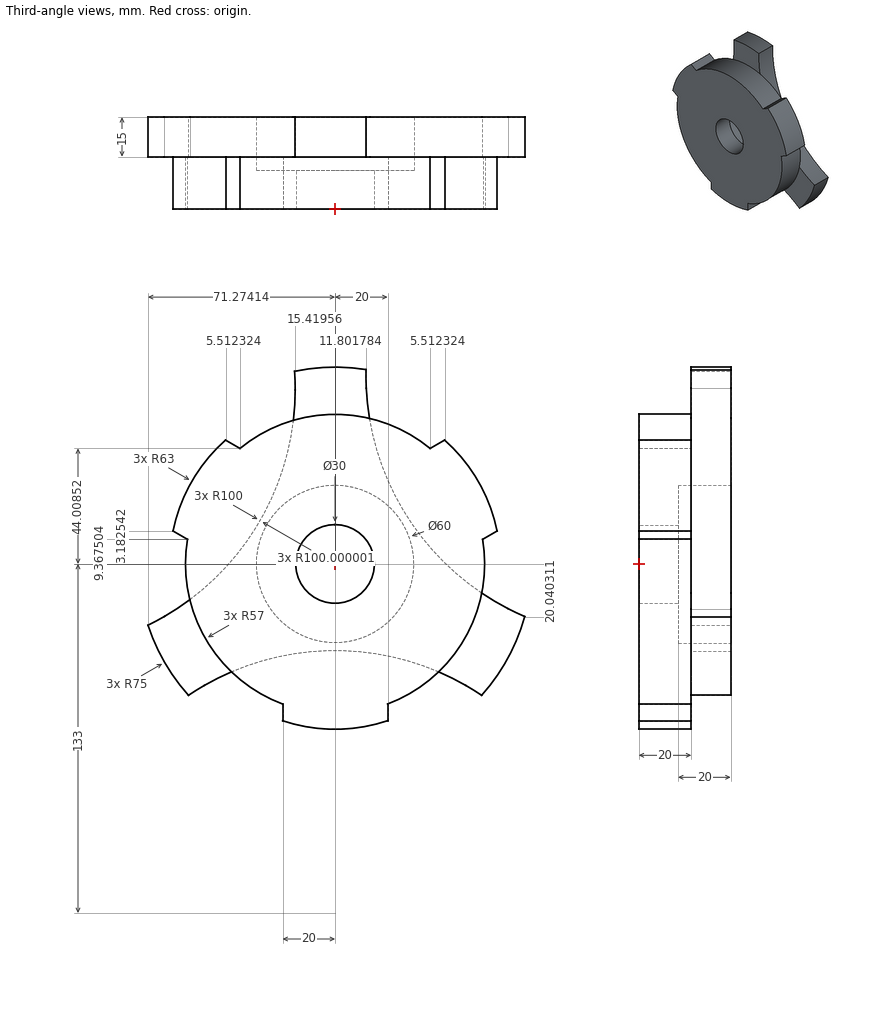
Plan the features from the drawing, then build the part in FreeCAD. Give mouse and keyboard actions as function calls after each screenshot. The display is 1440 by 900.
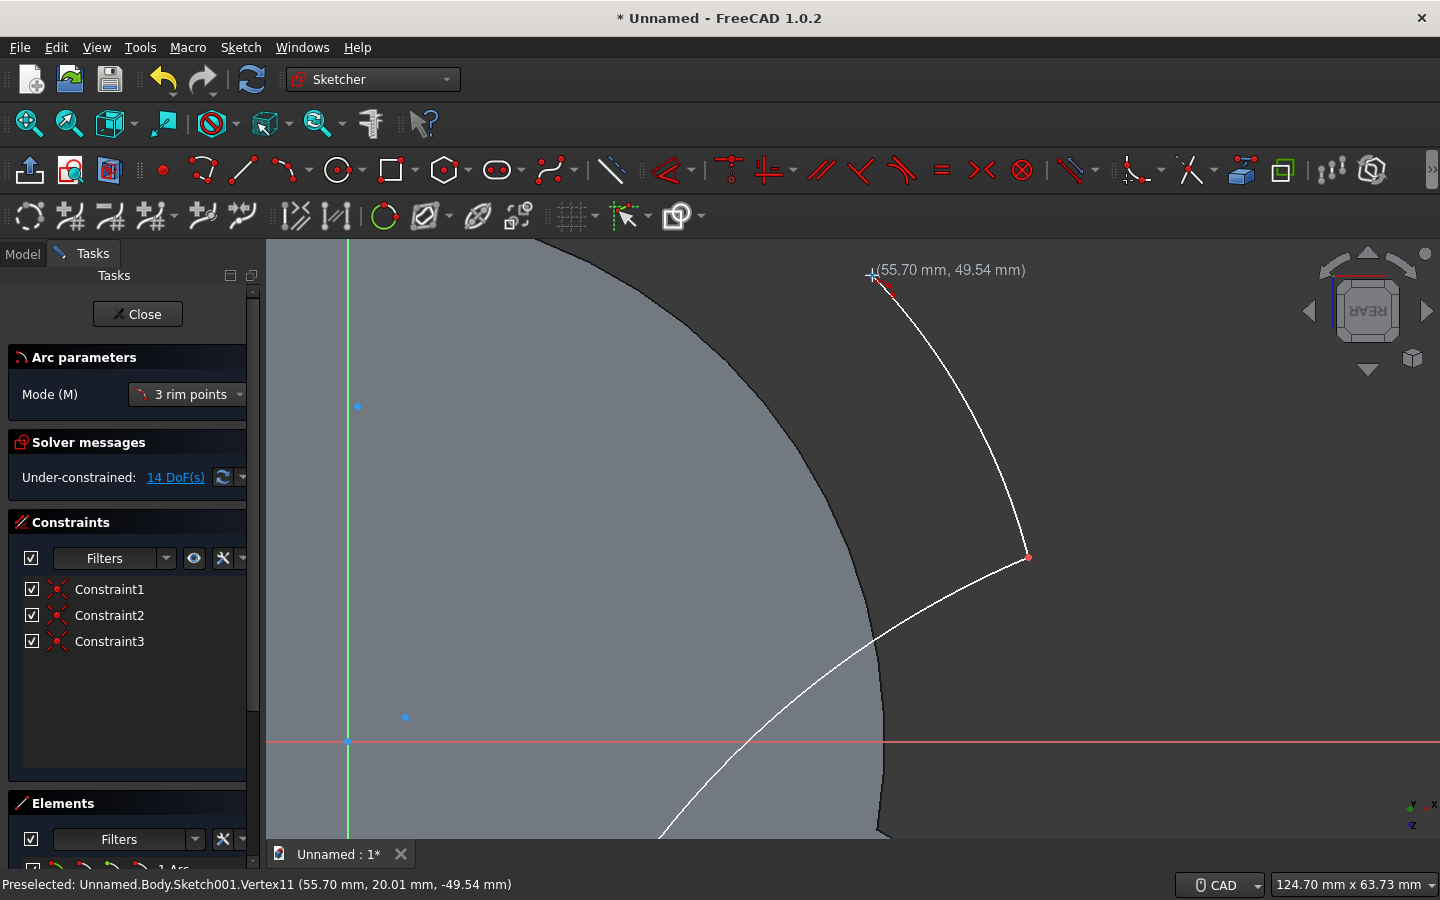
scroll(971, 401, down, 6)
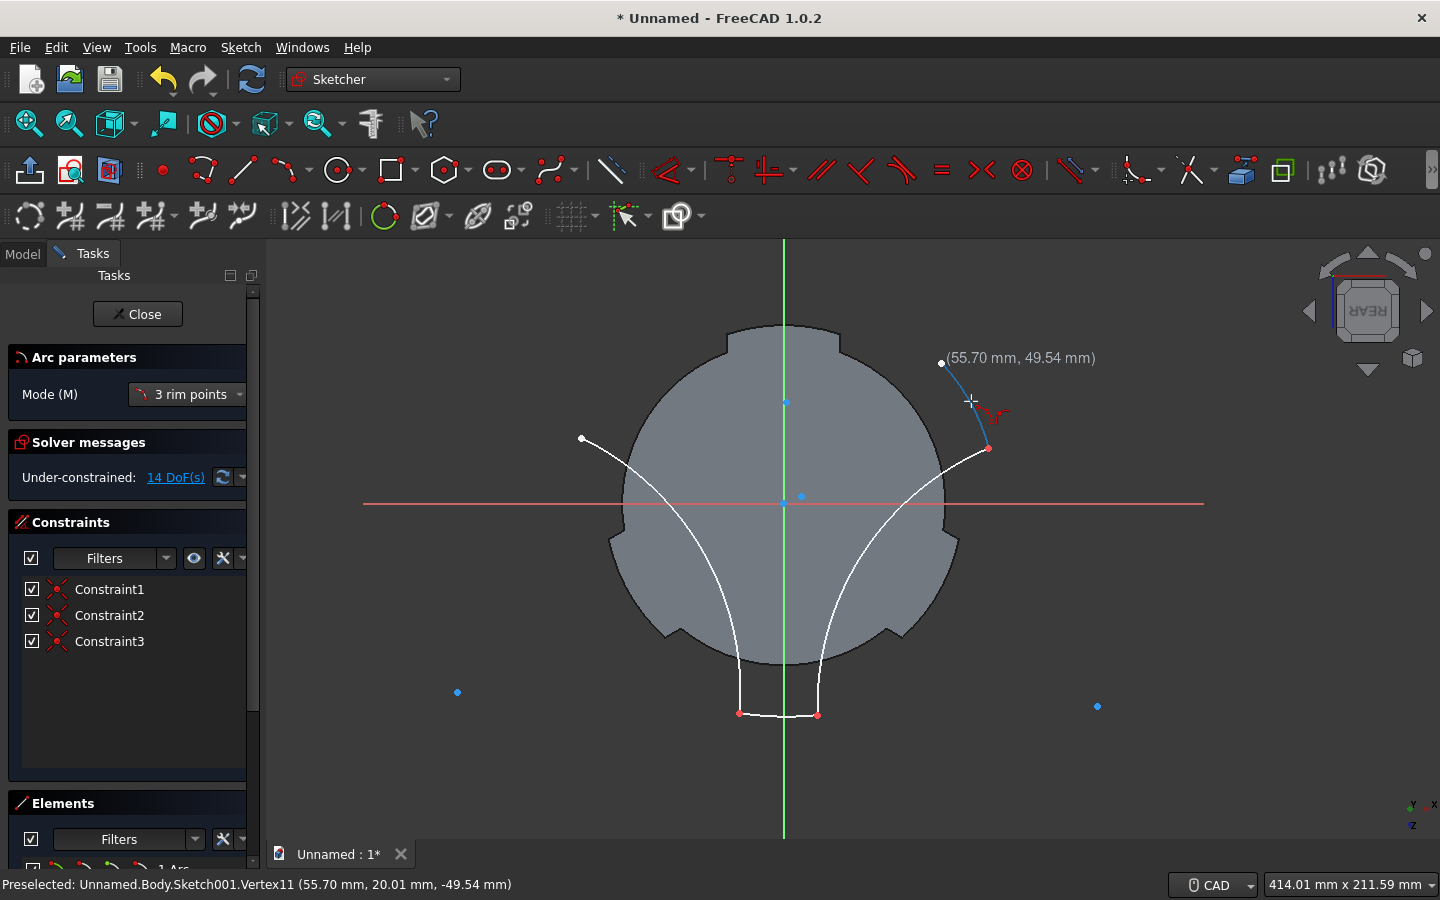
click(625, 362)
click(750, 408)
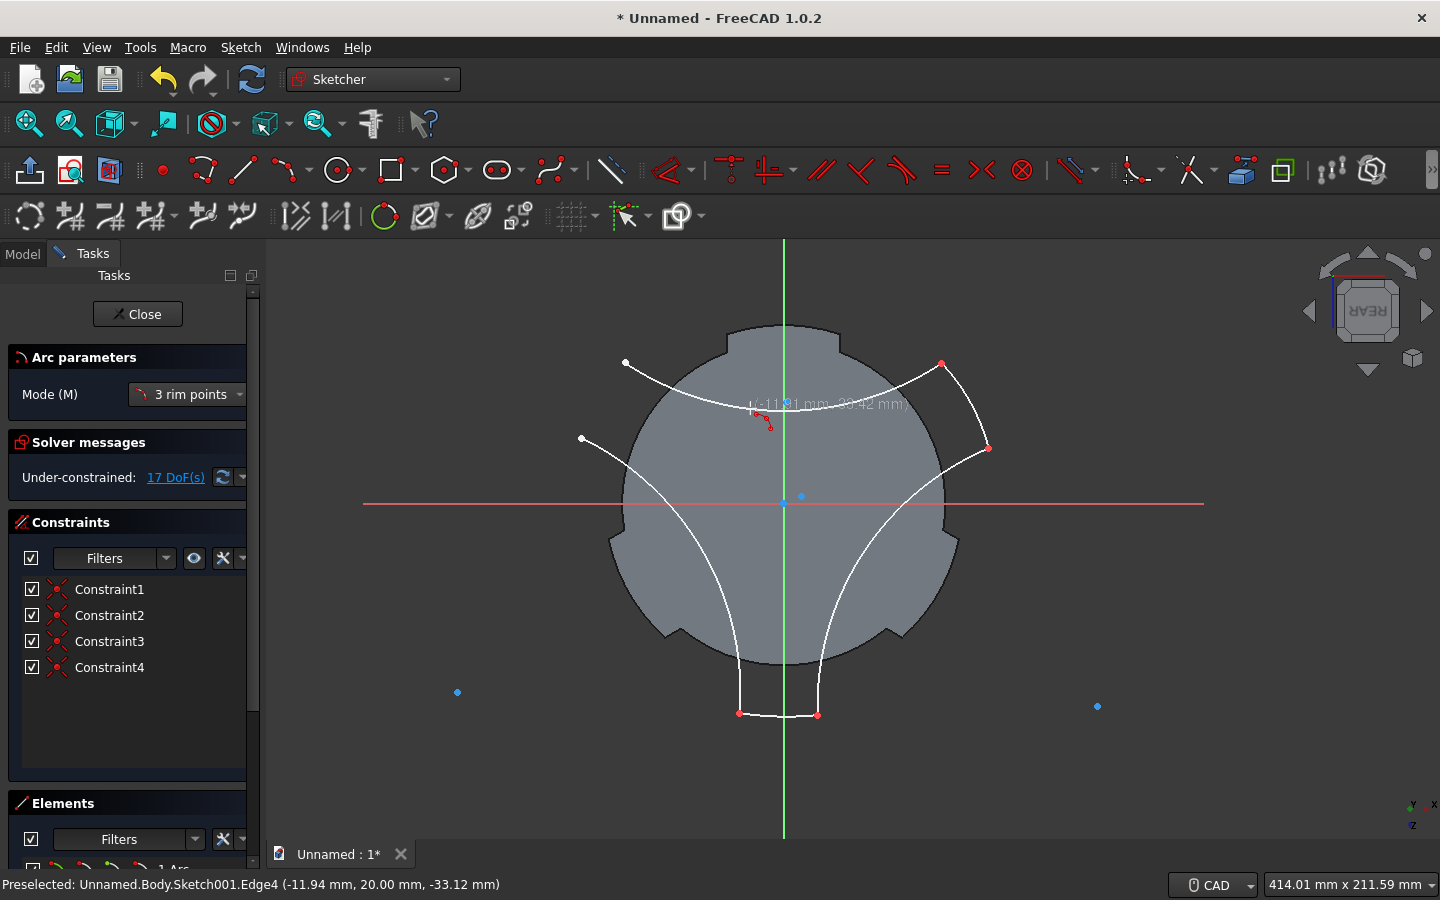
click(625, 363)
click(582, 438)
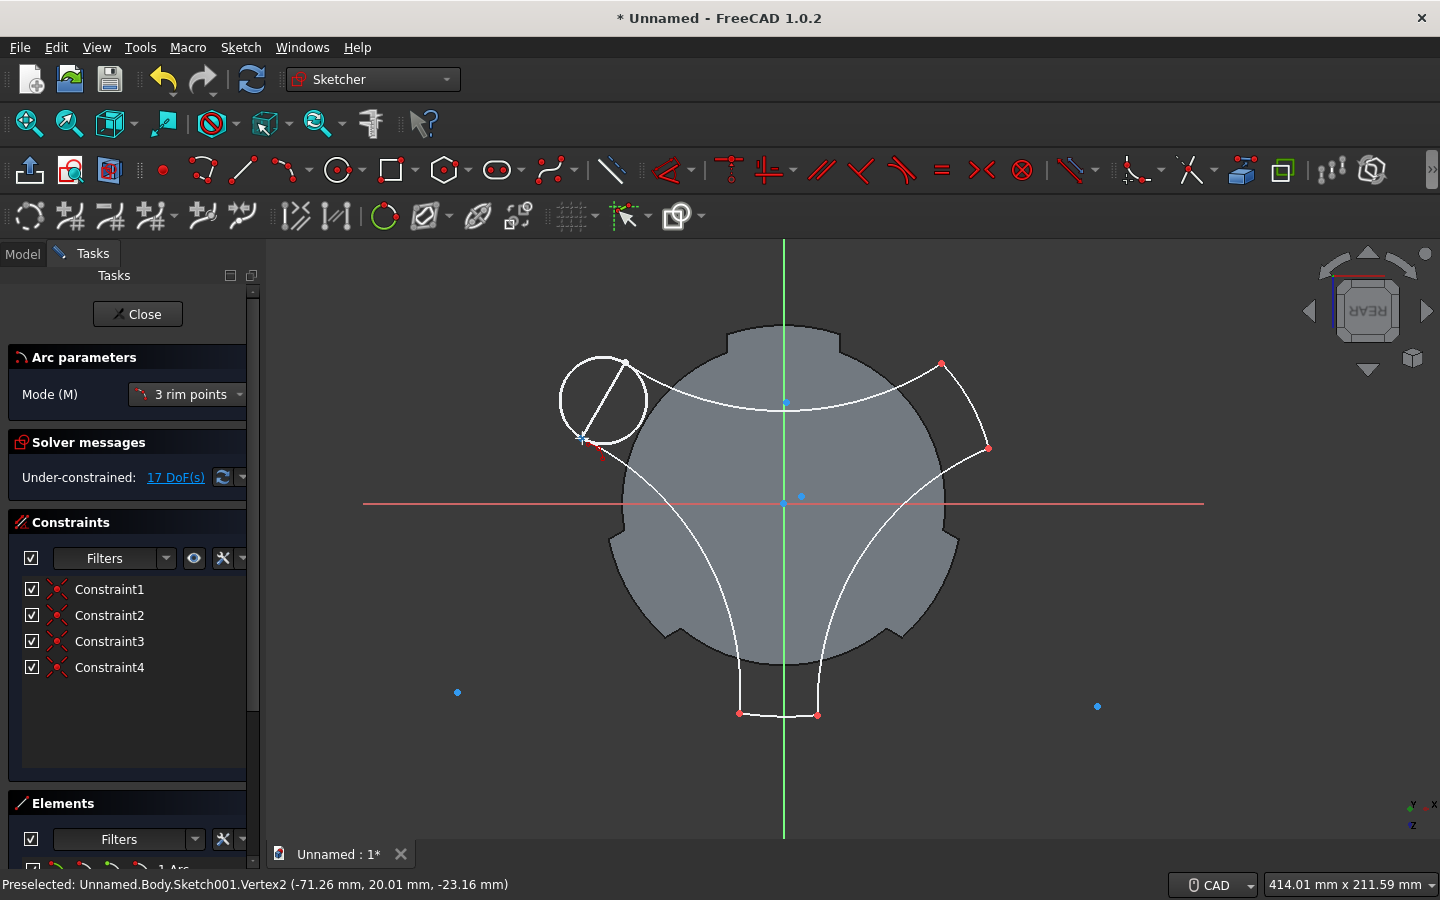
scroll(600, 397, up, 7)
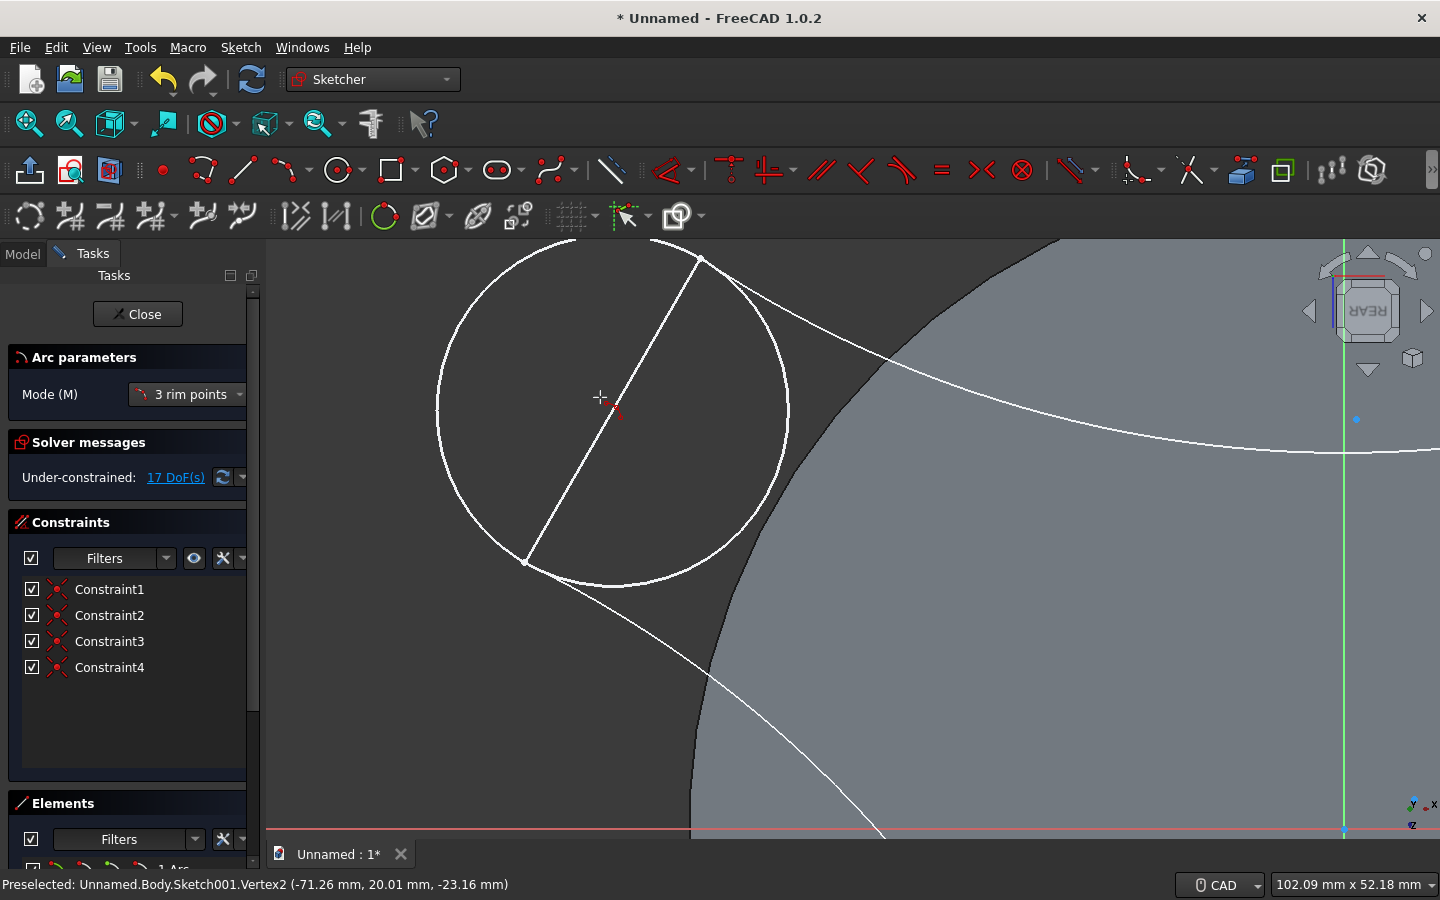
click(597, 398)
key(Escape)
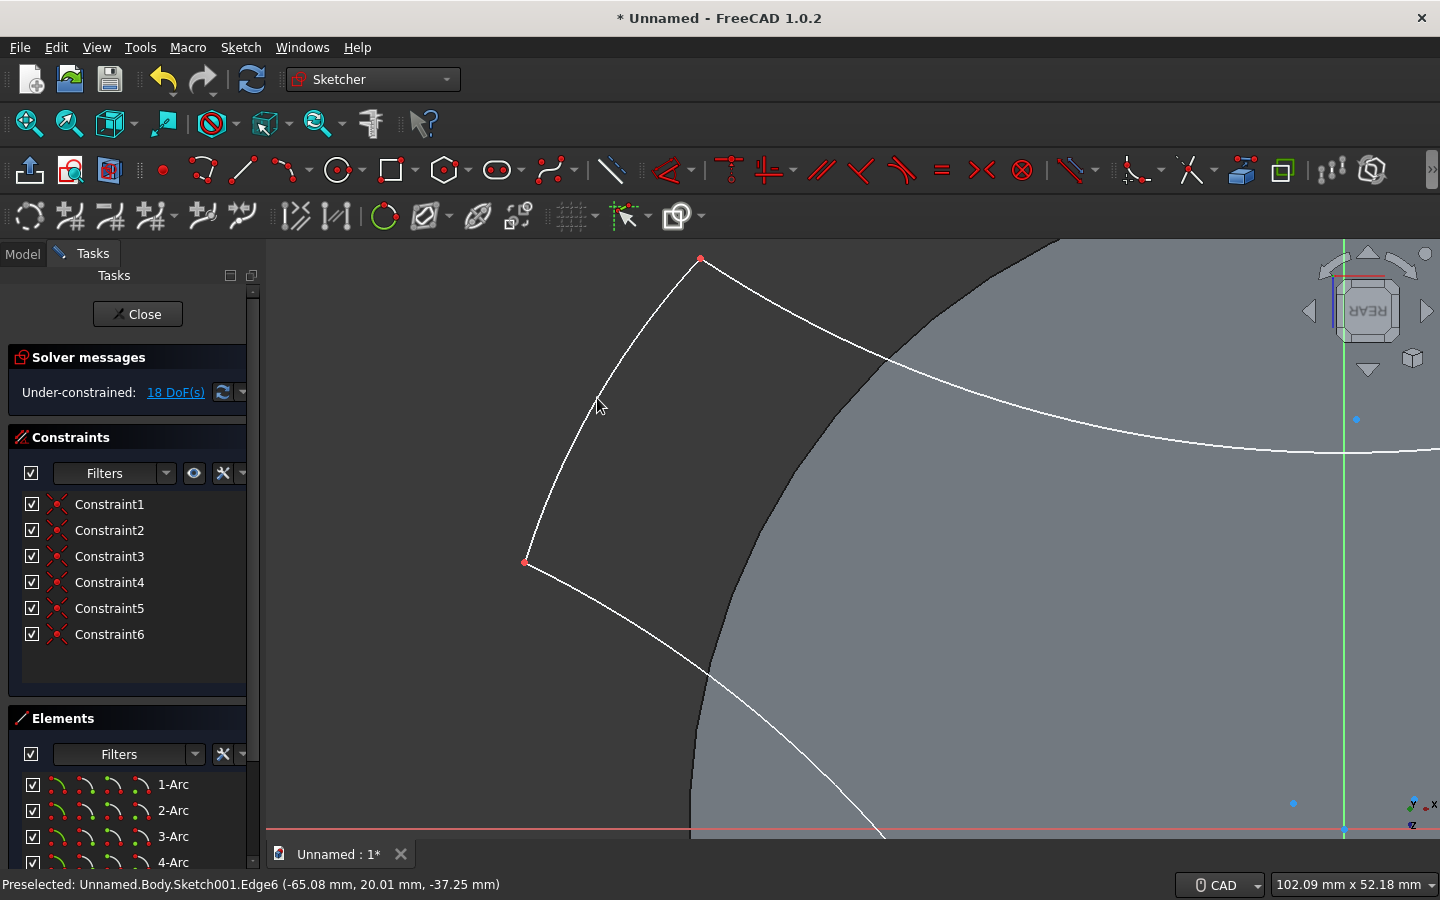
scroll(599, 397, down, 7)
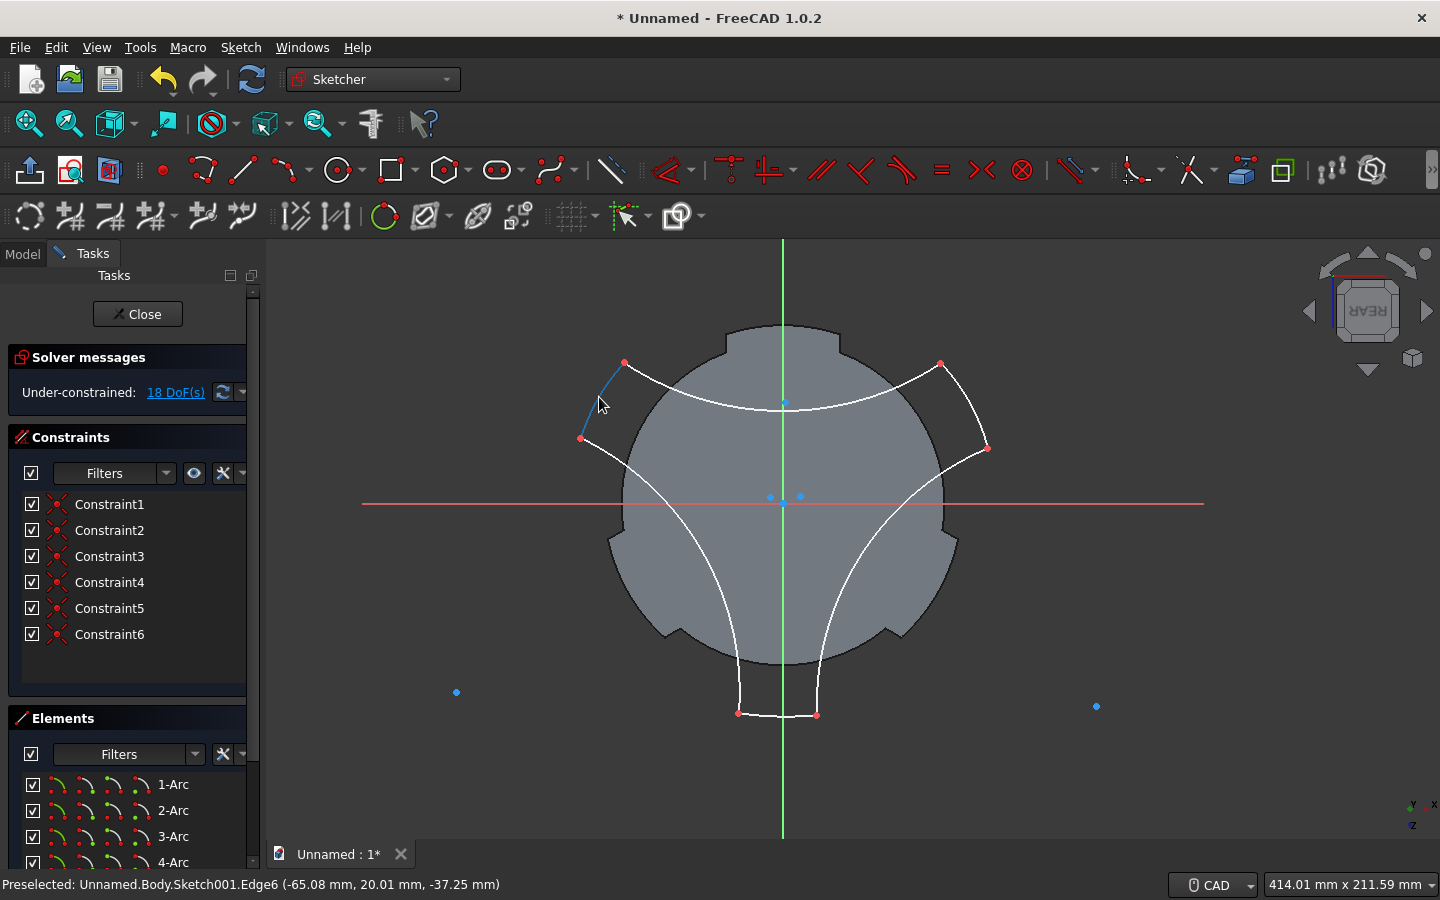
click(762, 716)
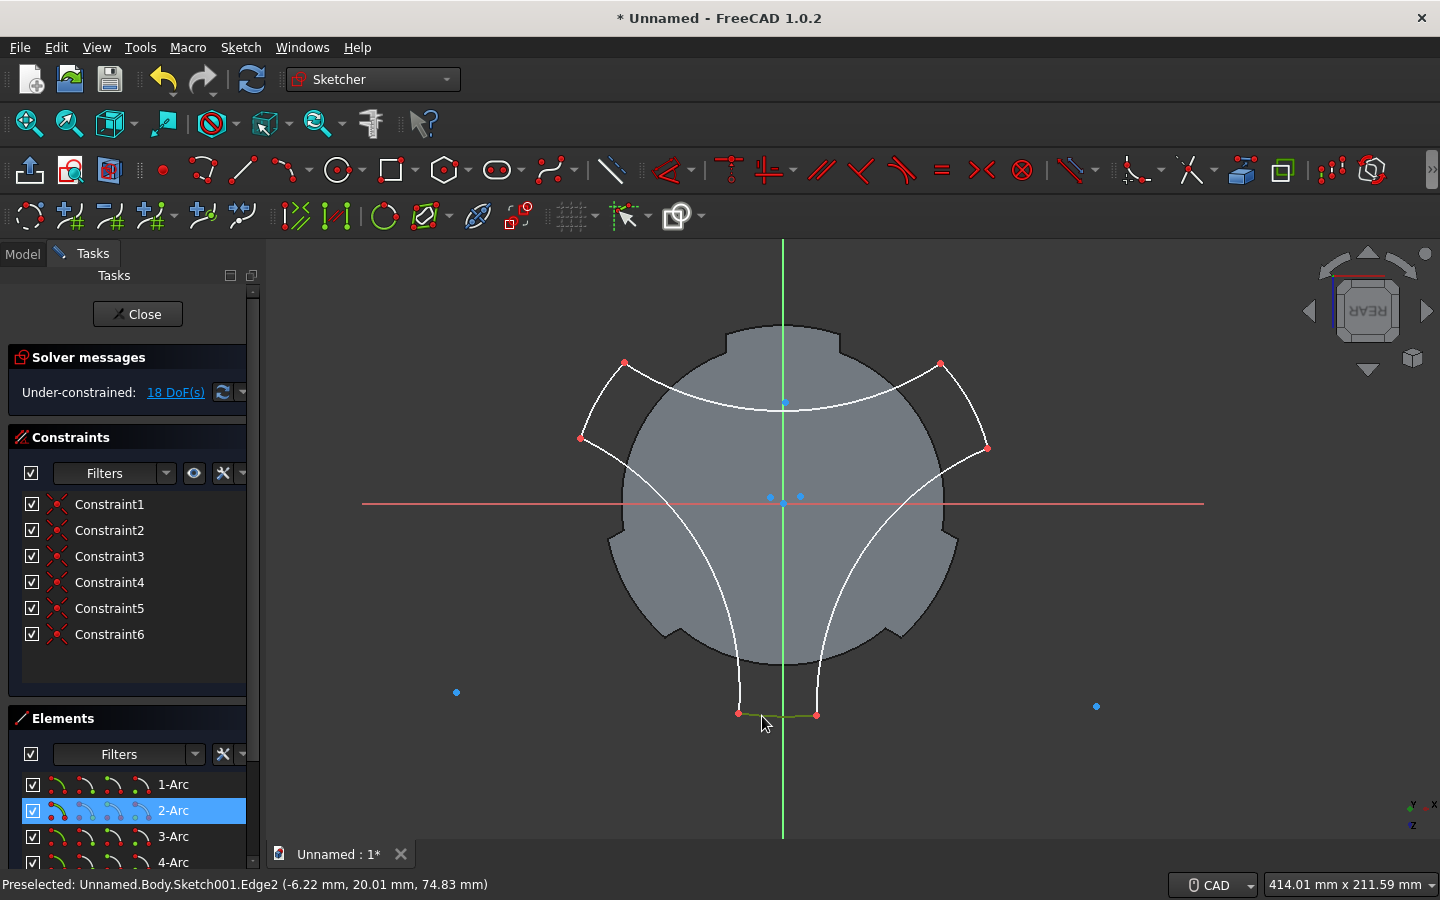
click(978, 420)